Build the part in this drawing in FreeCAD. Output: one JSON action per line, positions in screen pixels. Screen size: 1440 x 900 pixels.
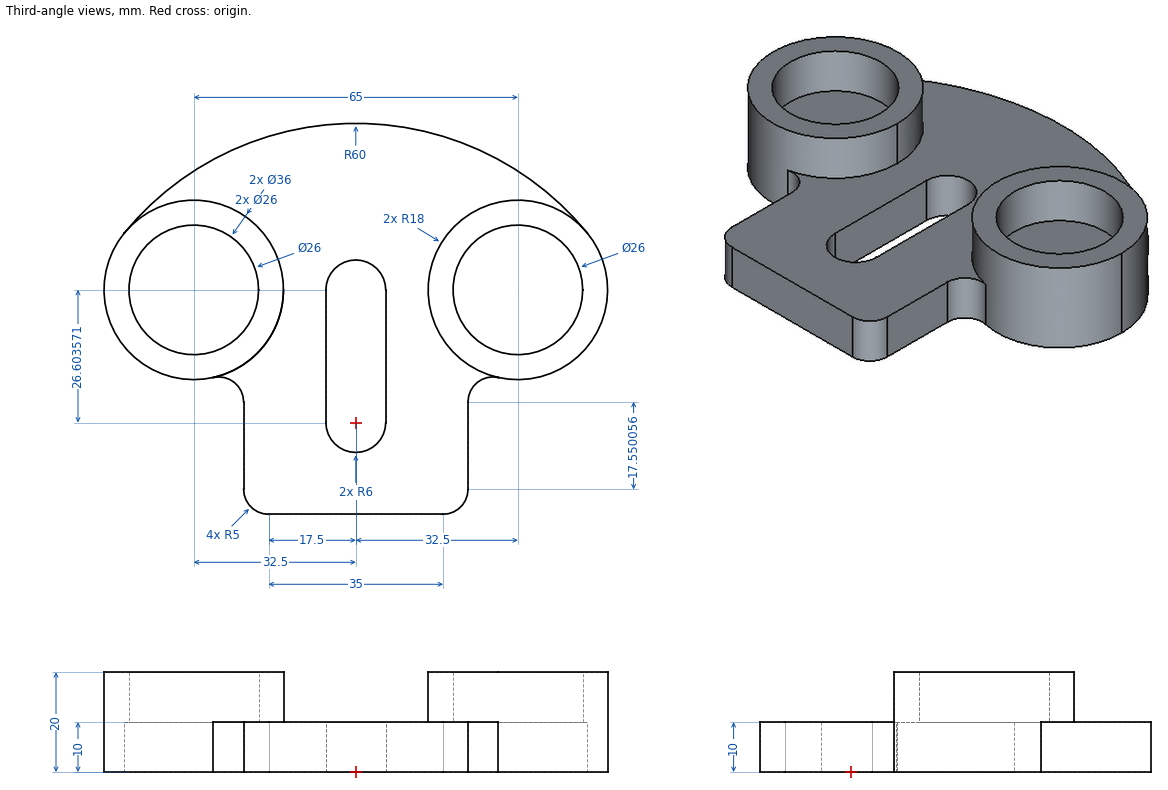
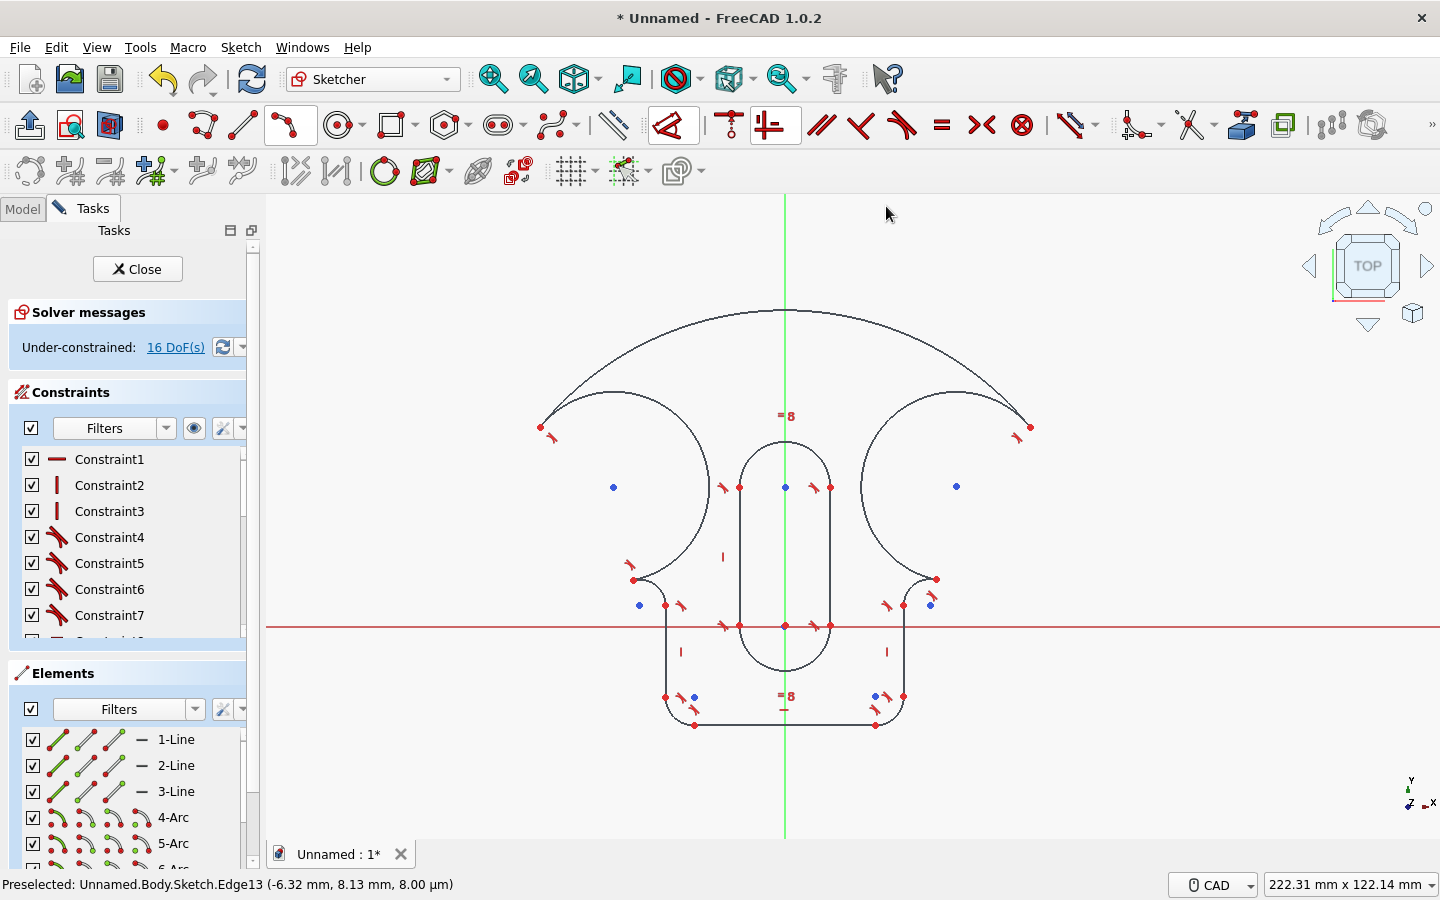
{"action": "scroll", "coordinate": [785, 626], "scroll_direction": "up", "scroll_amount": 3}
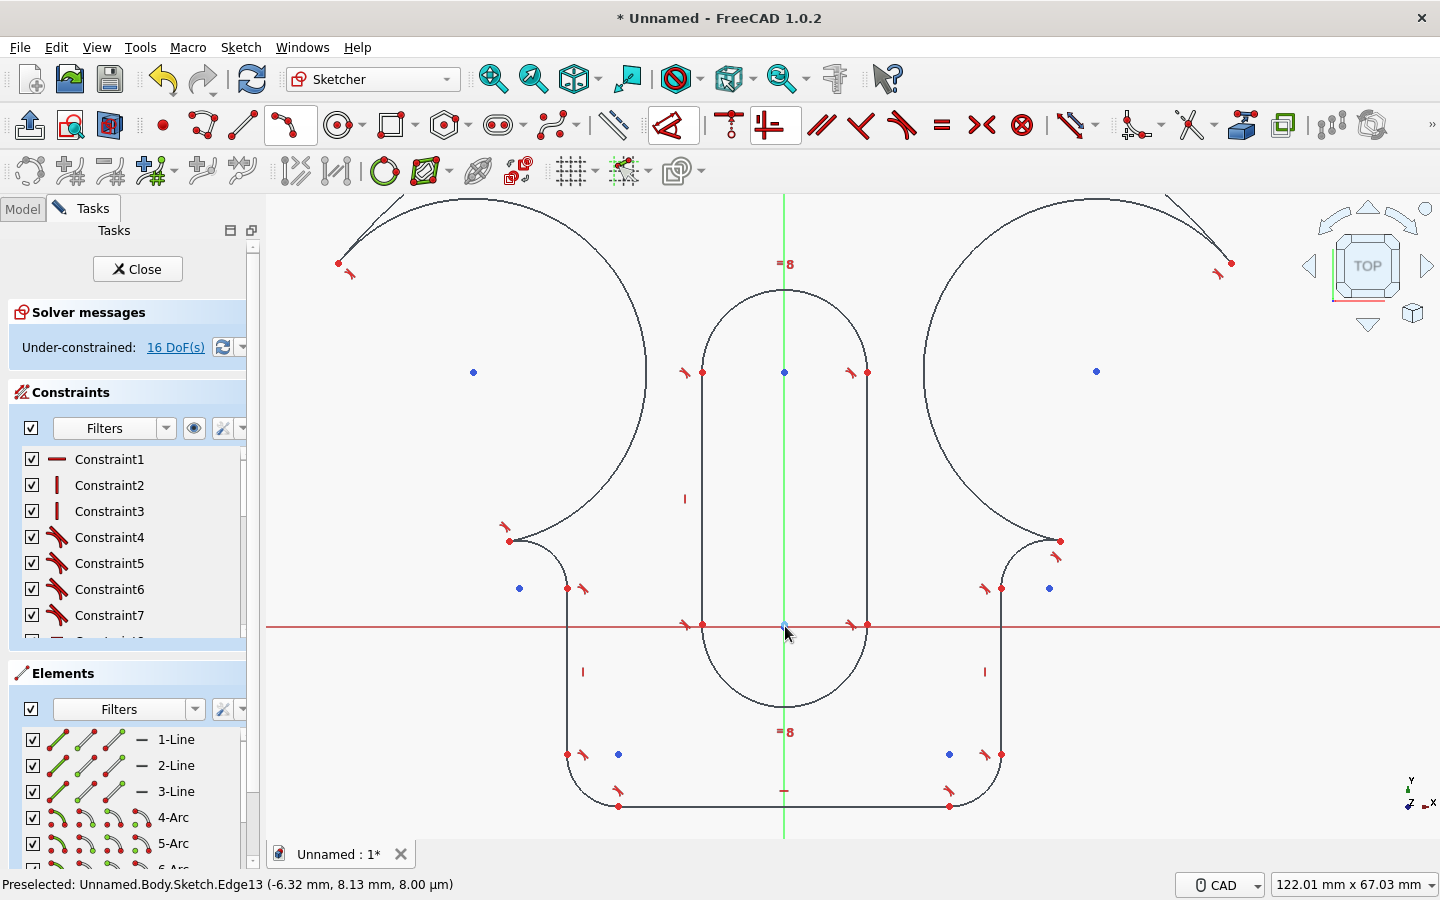
{"action": "left_click_drag", "start_coordinate": [774, 615], "coordinate": [795, 637]}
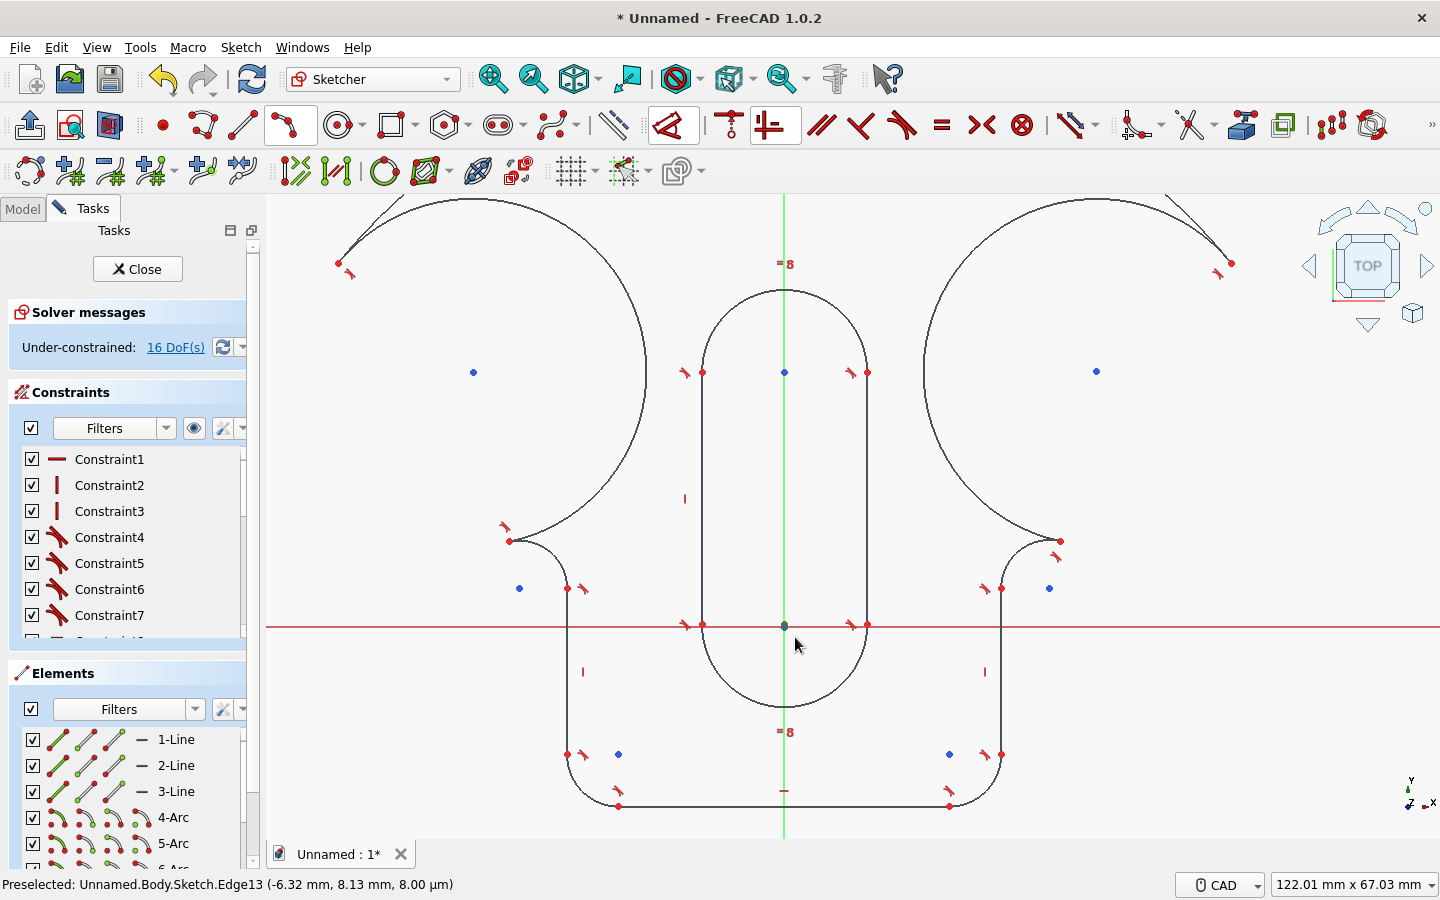
{"action": "left_click", "coordinate": [730, 126]}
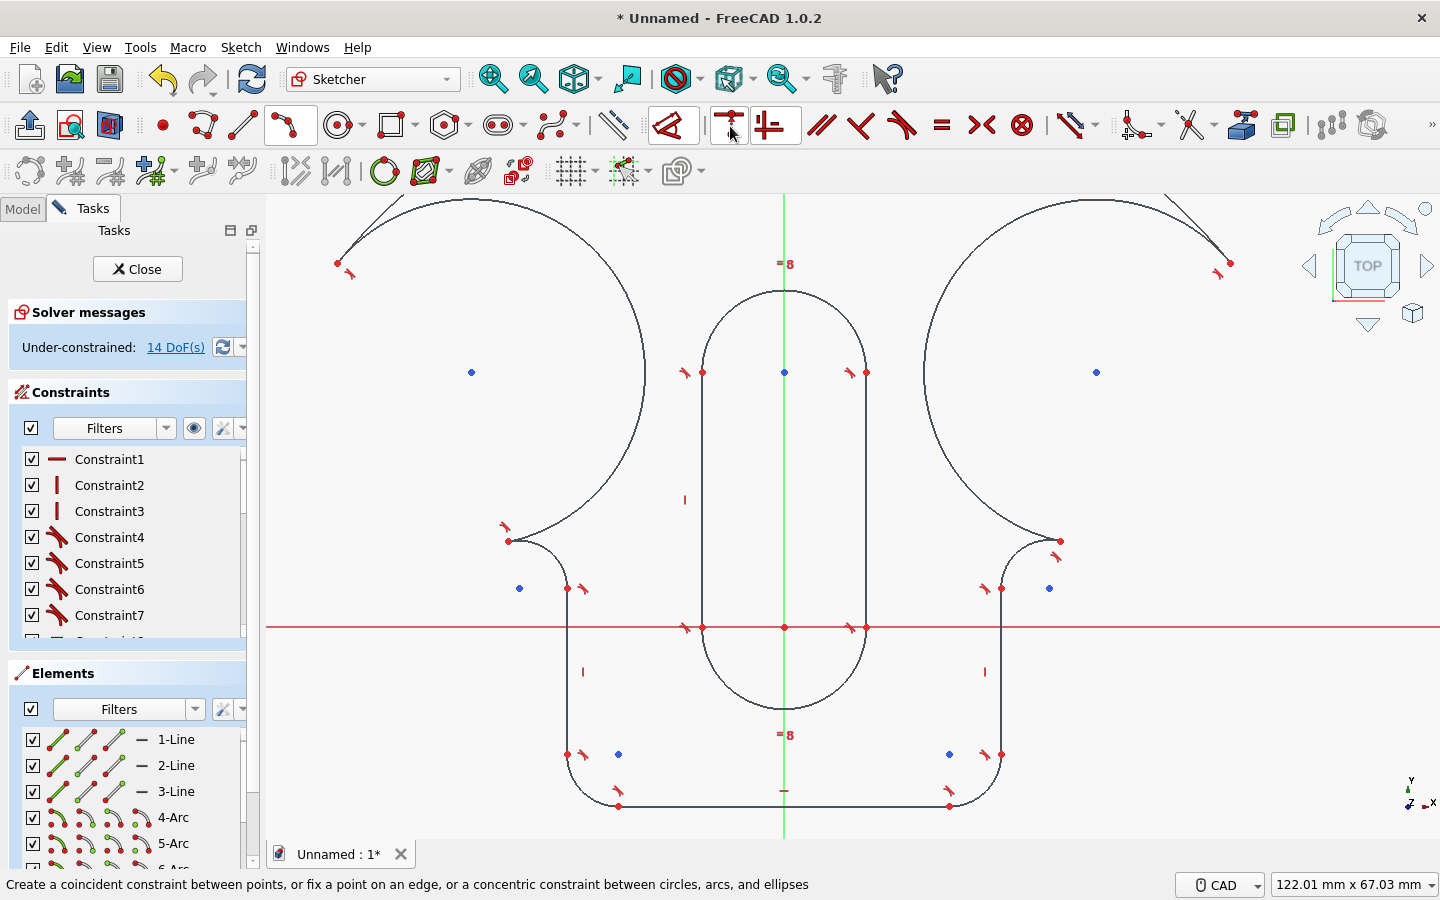
{"action": "left_click", "coordinate": [973, 801]}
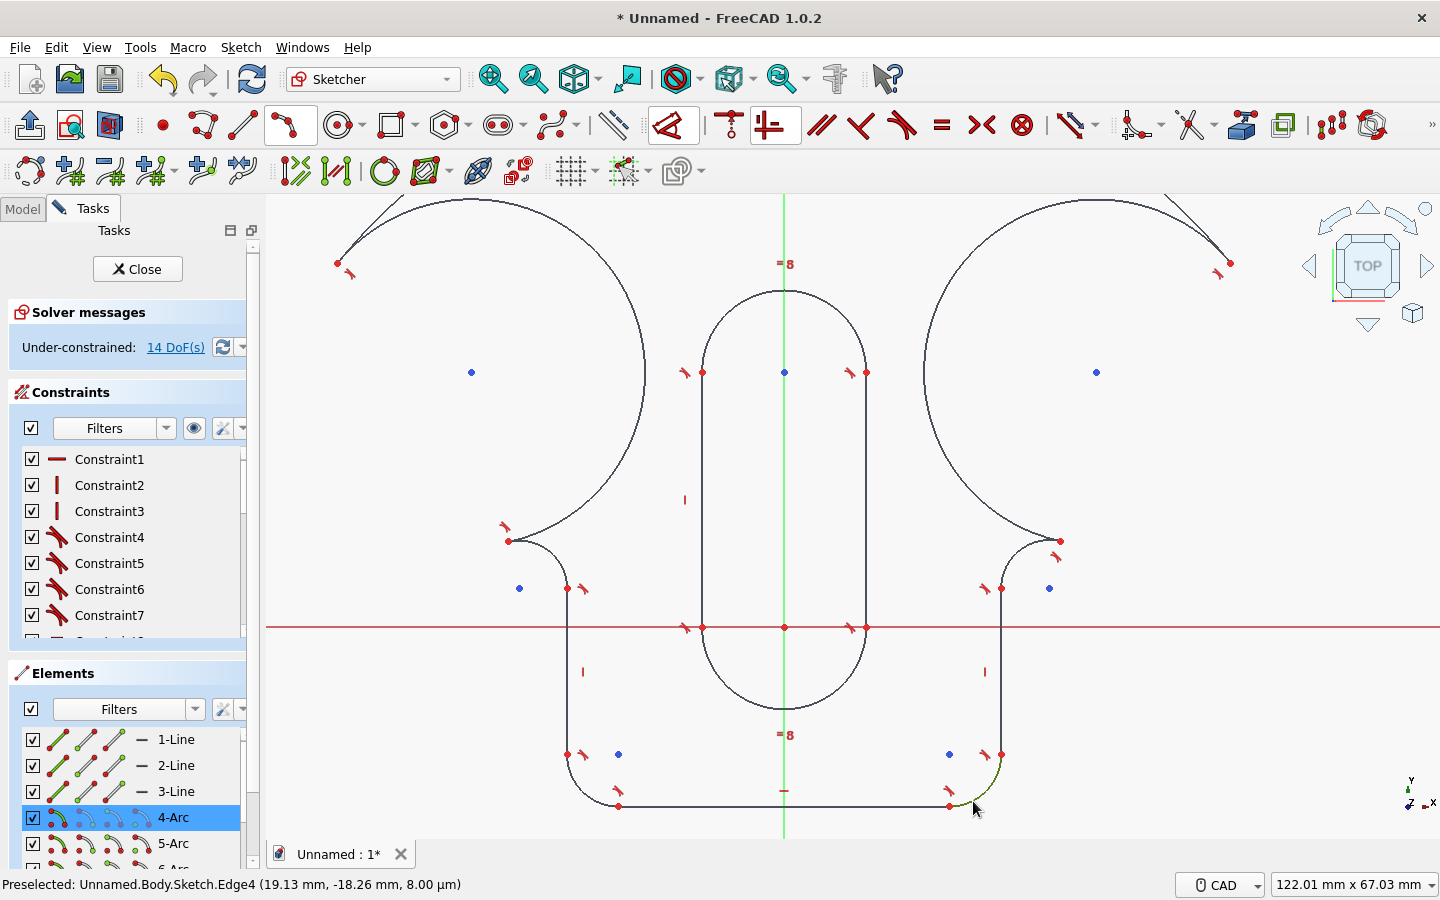
{"action": "left_click", "coordinate": [1008, 564]}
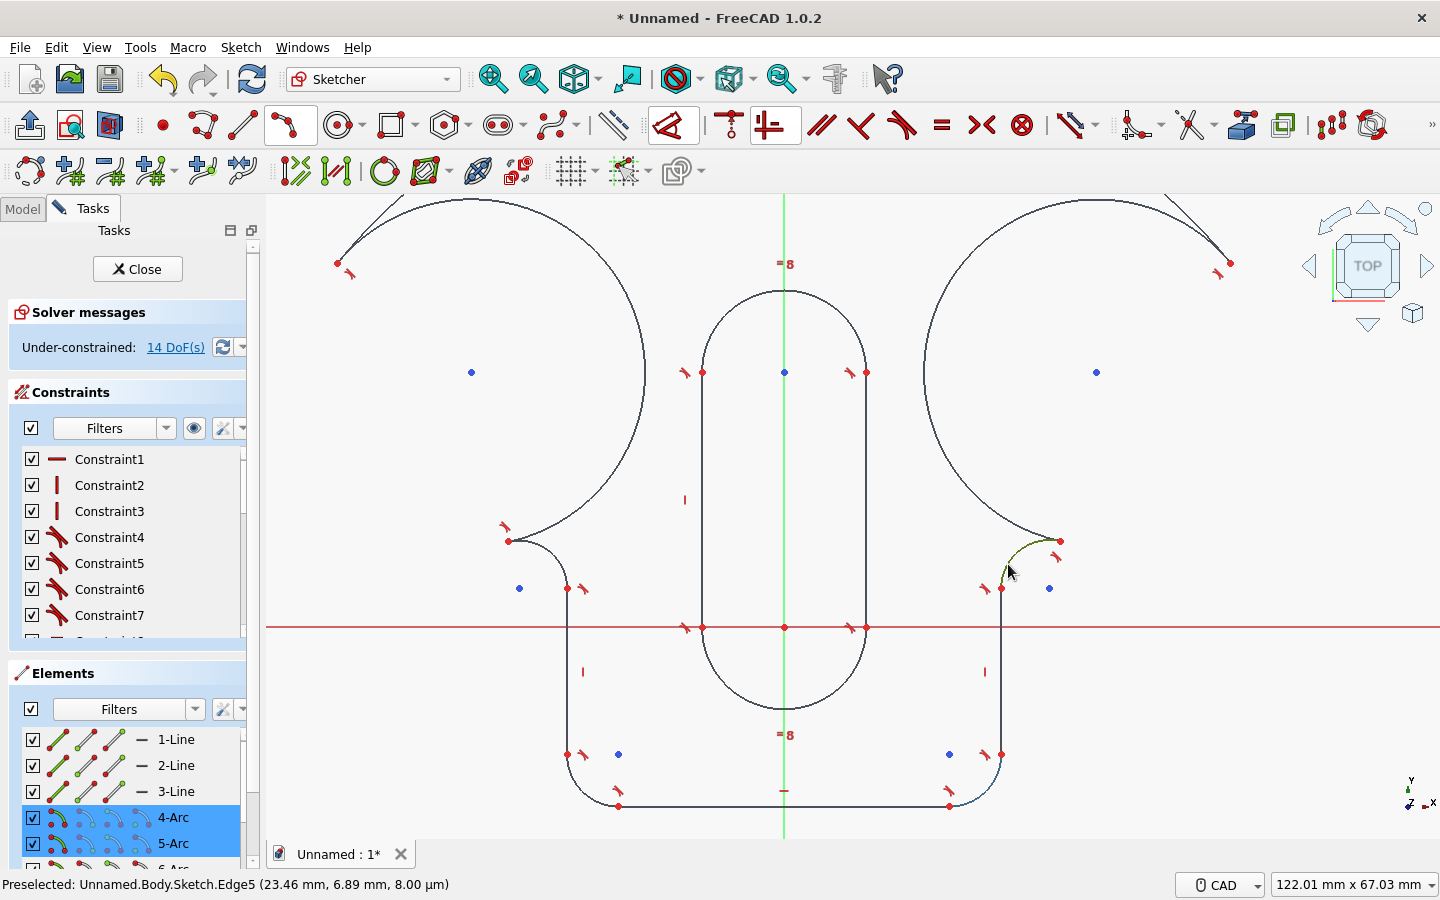
{"action": "left_click", "coordinate": [560, 564]}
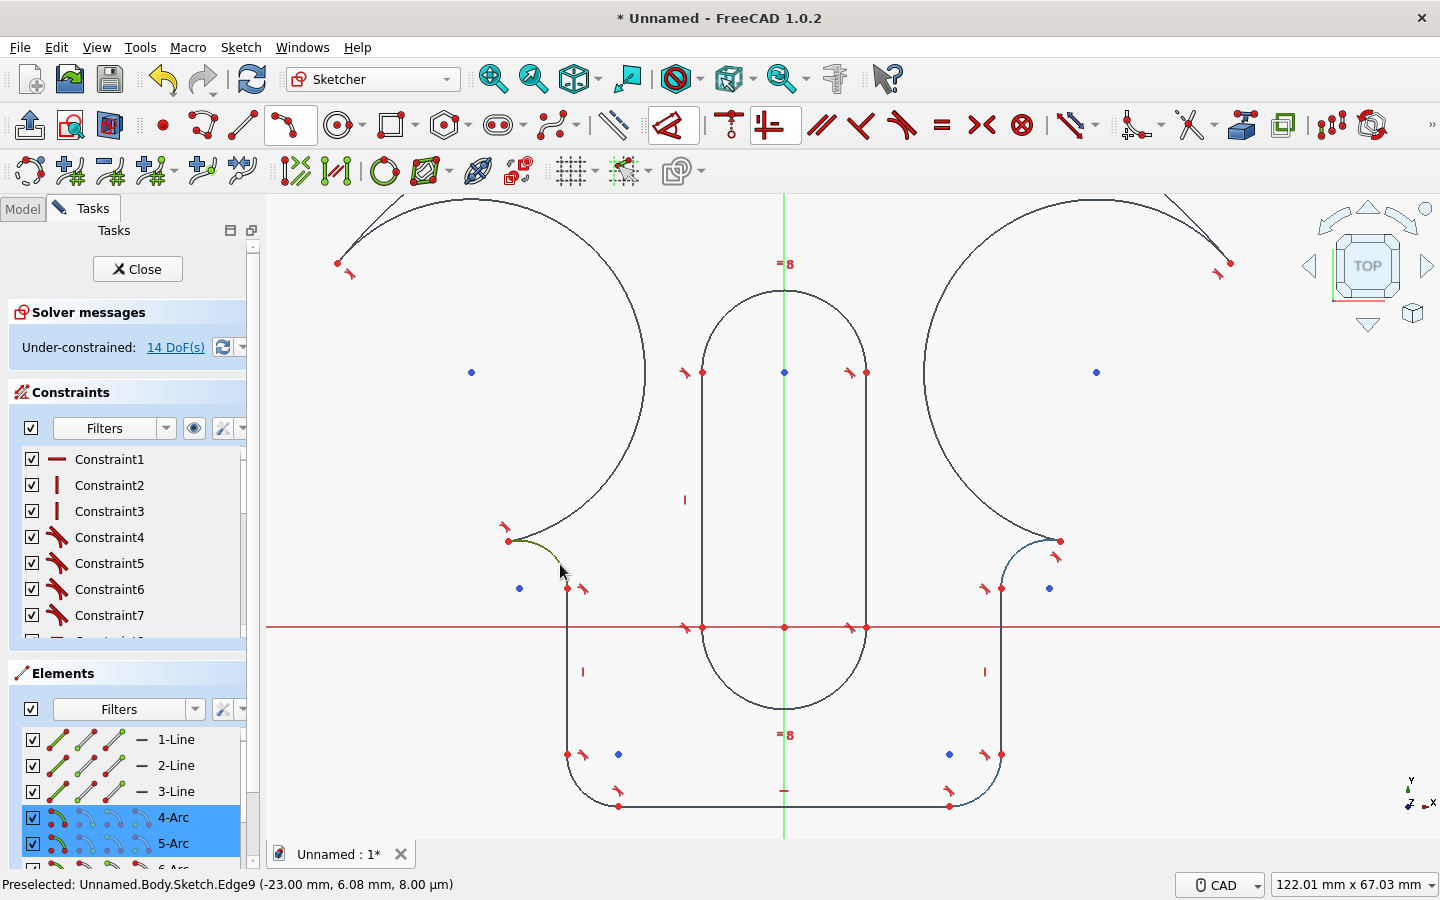
{"action": "left_click", "coordinate": [573, 778]}